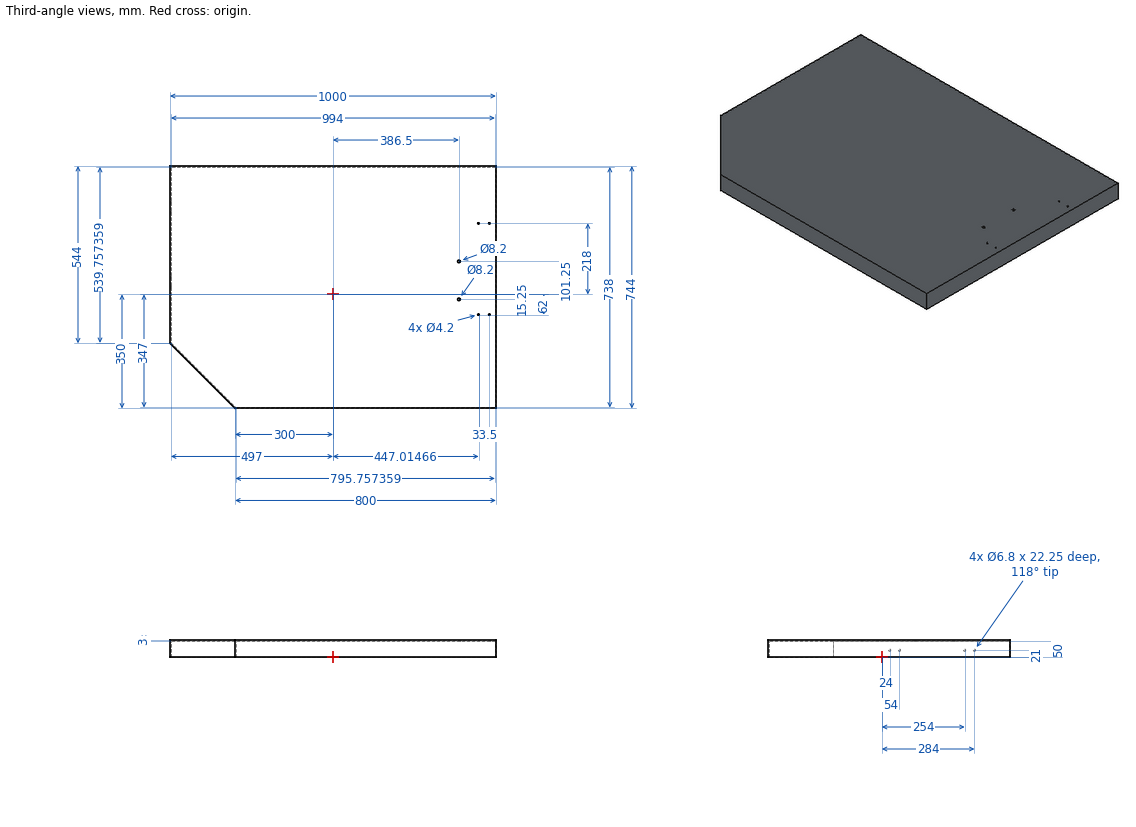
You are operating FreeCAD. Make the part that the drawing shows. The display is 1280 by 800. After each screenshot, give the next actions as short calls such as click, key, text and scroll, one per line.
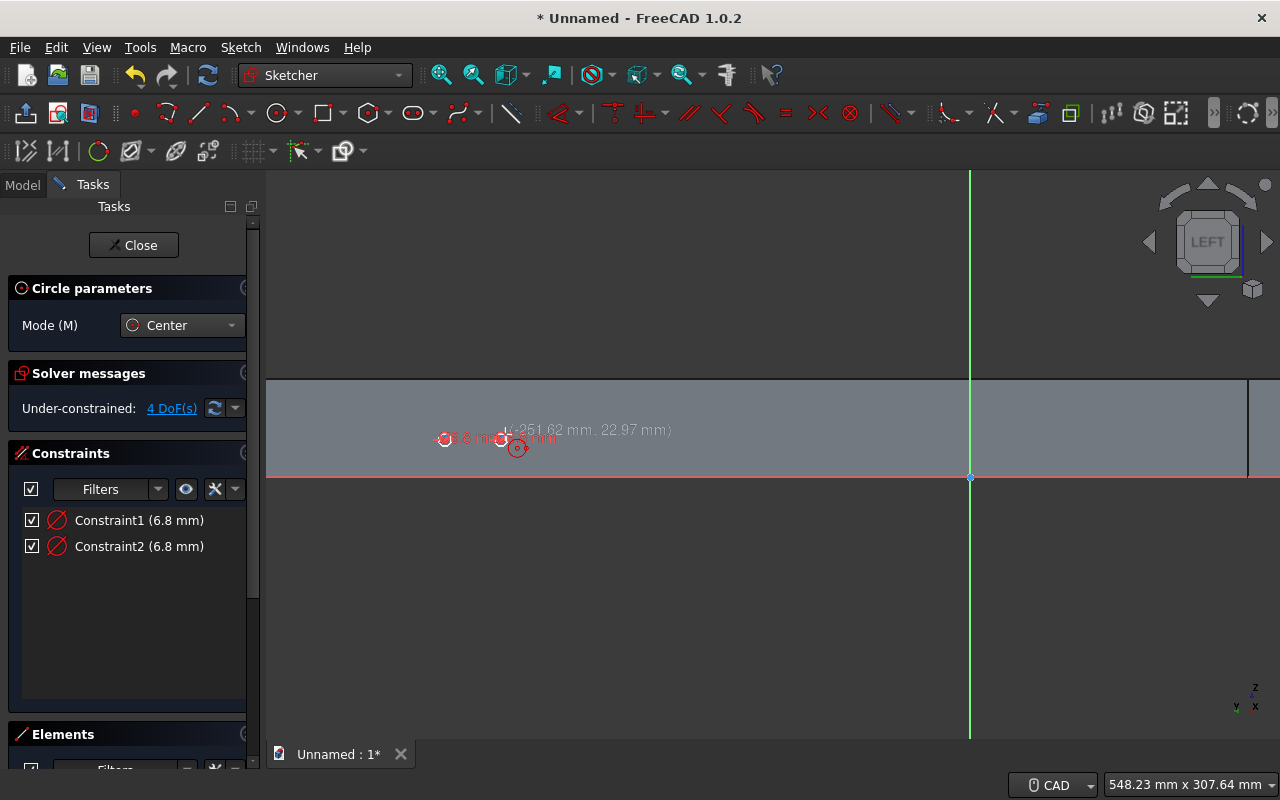
scroll(871, 439, up, 7)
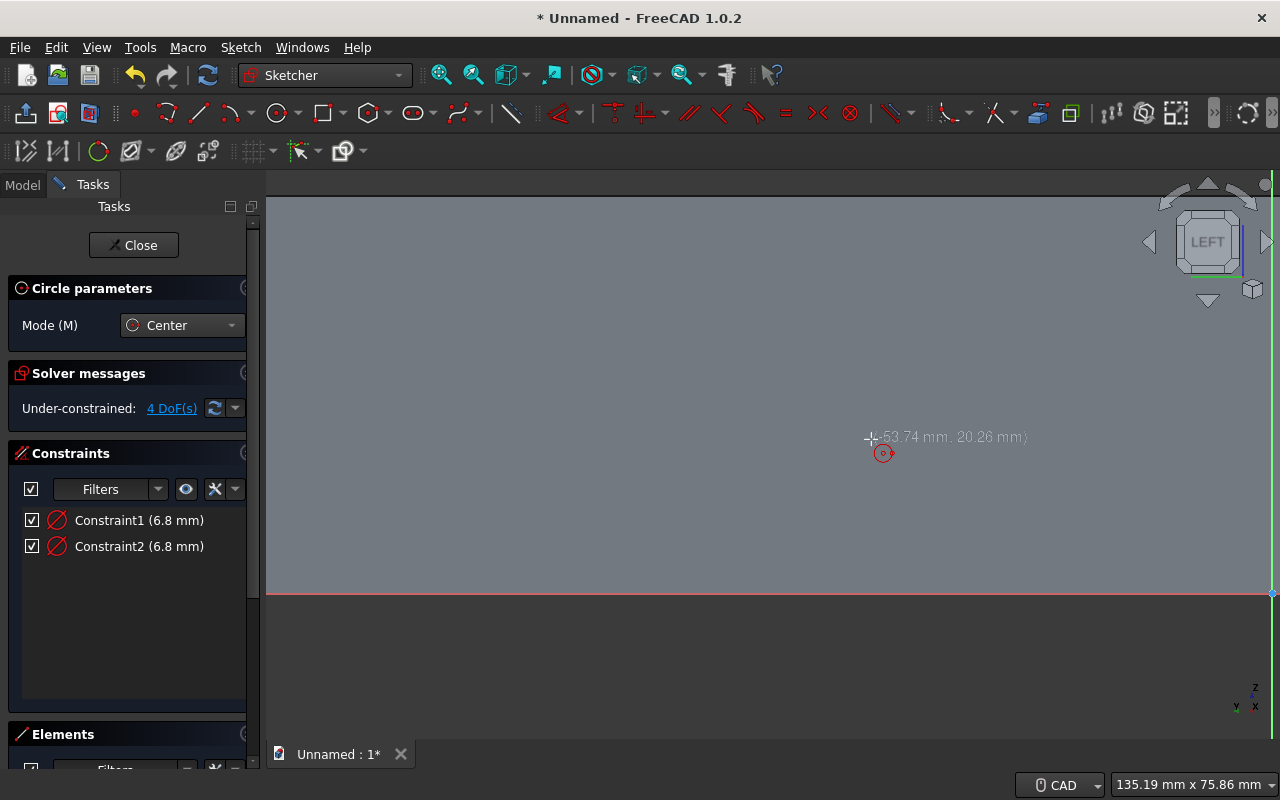
scroll(871, 439, down, 7)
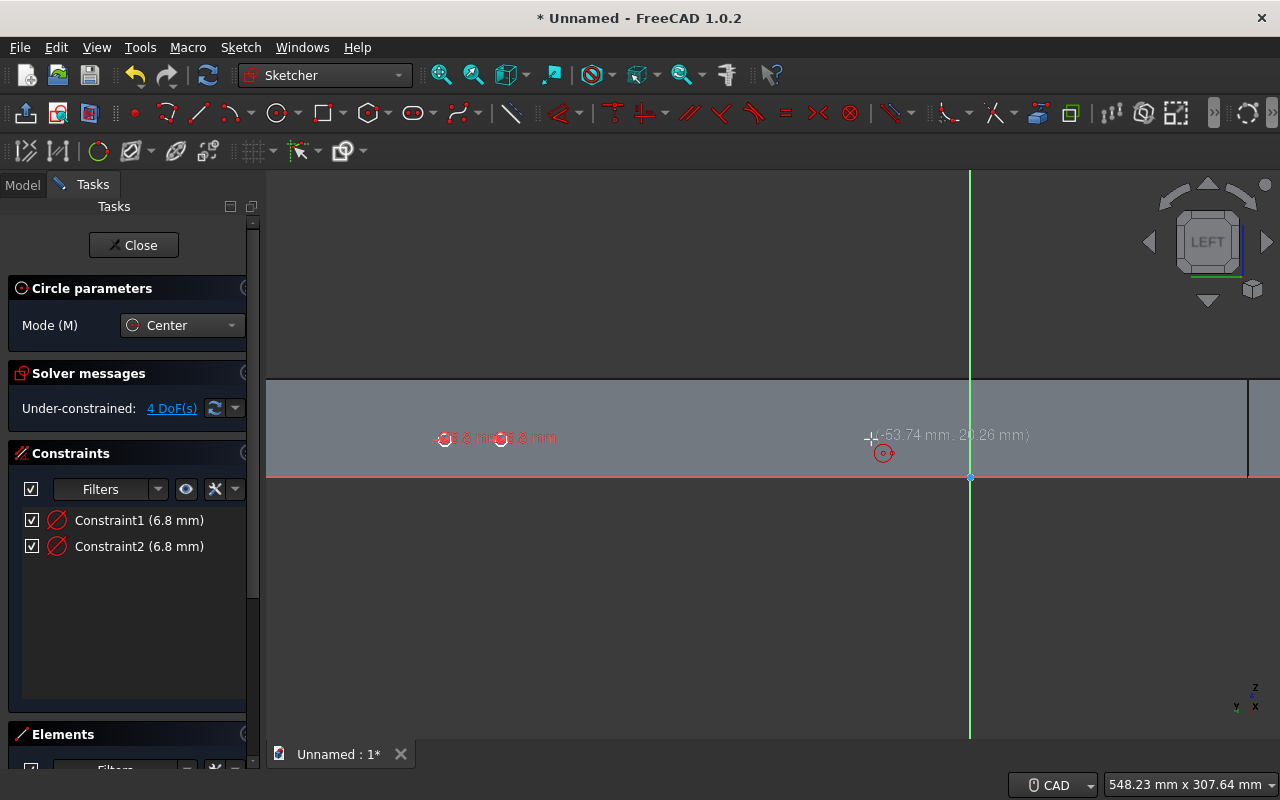
click(871, 439)
move(875, 434)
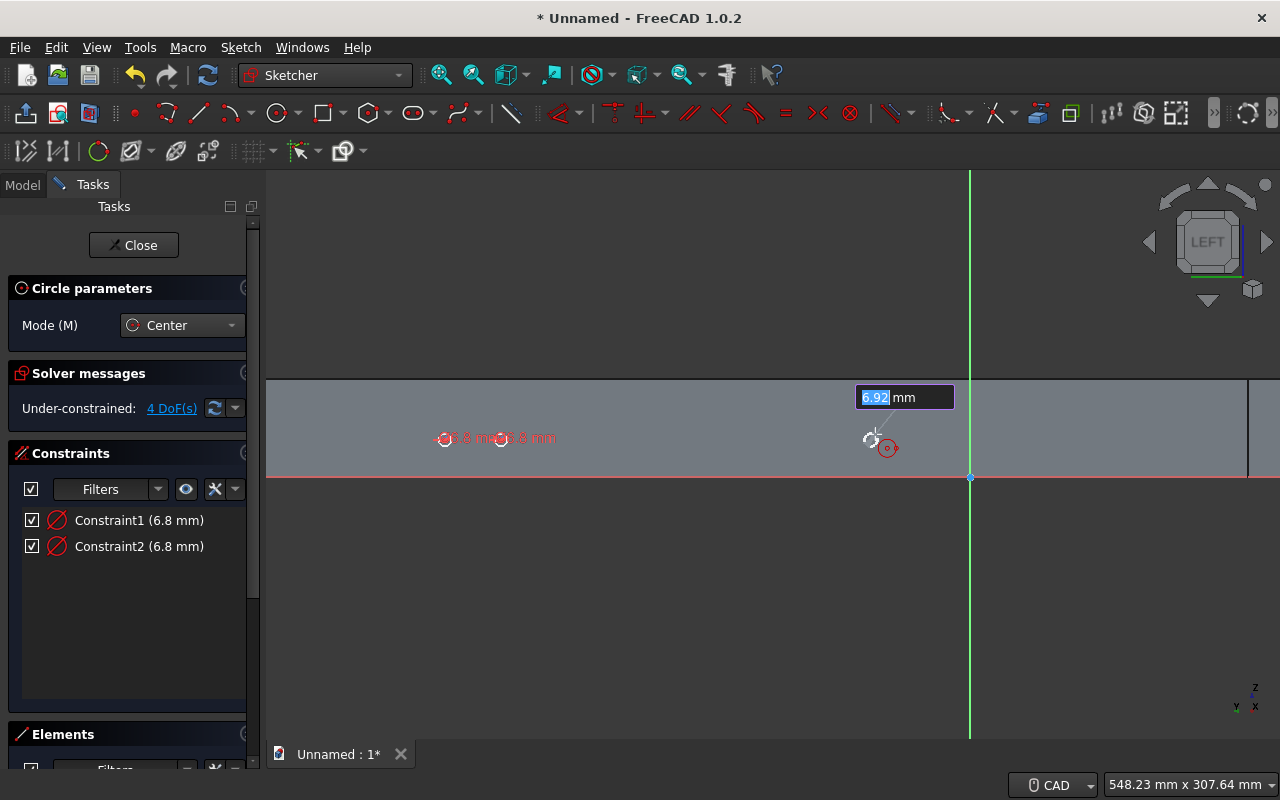
text(6.8)
key(Return)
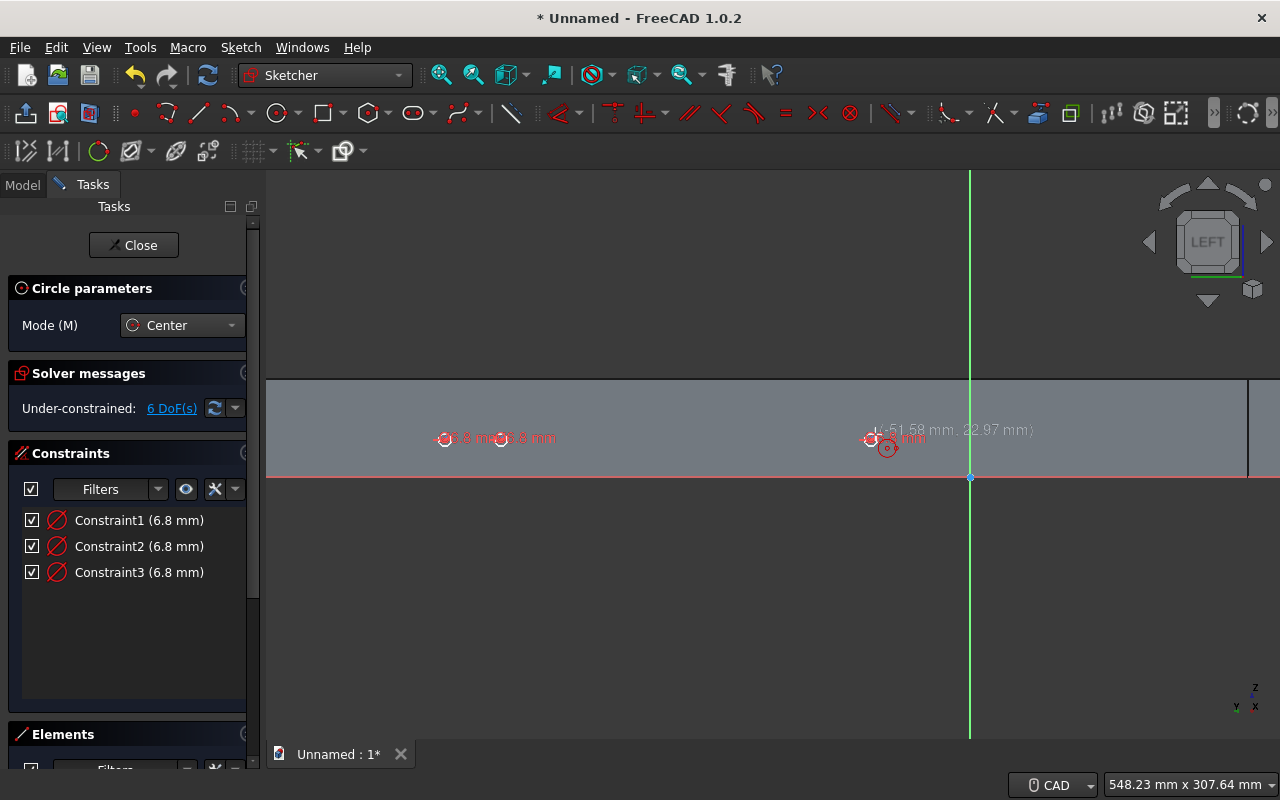
scroll(926, 439, up, 7)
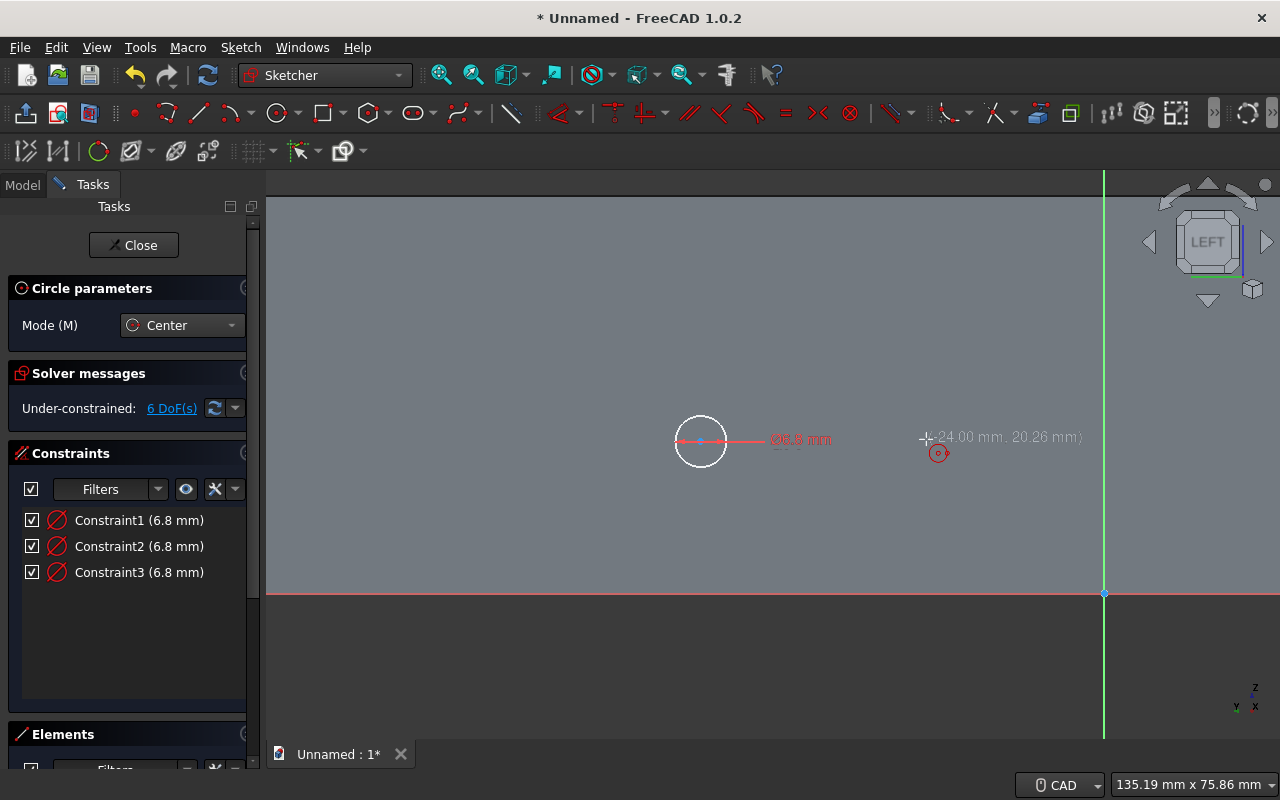
scroll(927, 439, down, 7)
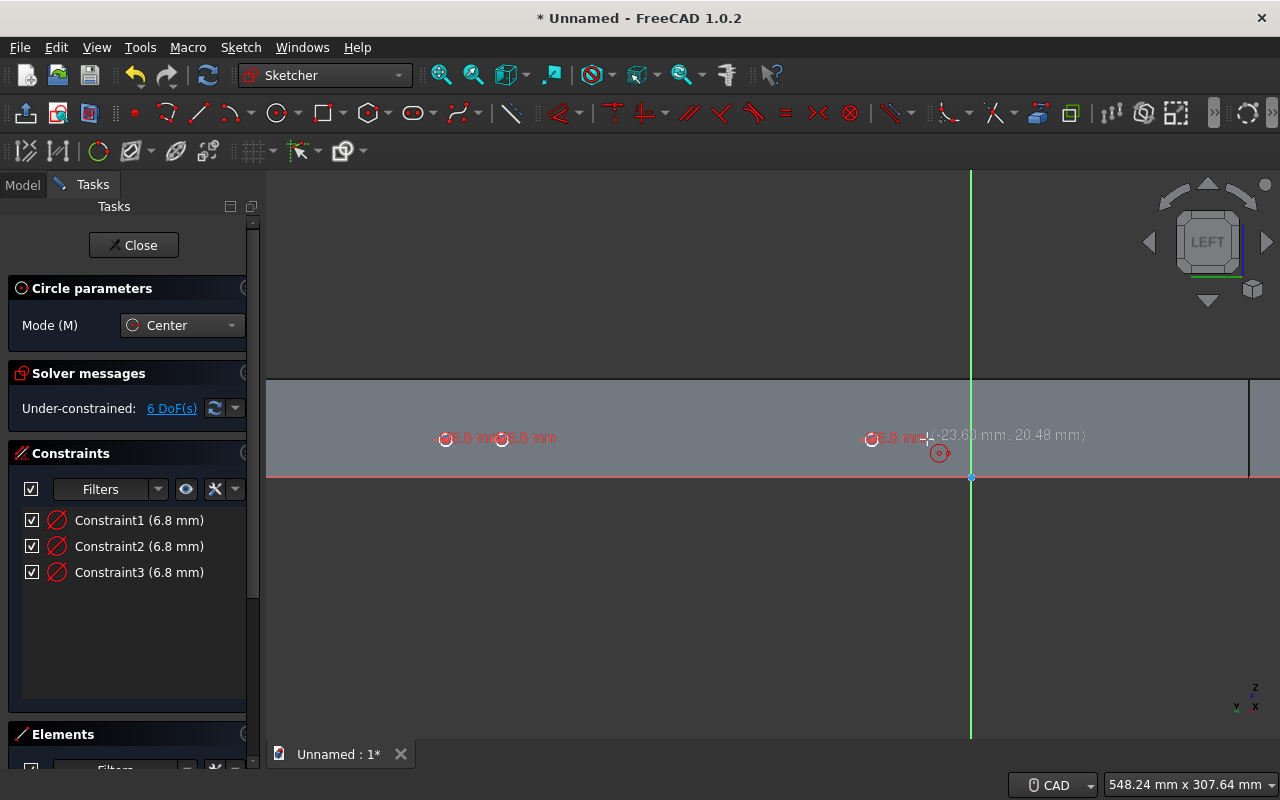
click(927, 439)
move(931, 434)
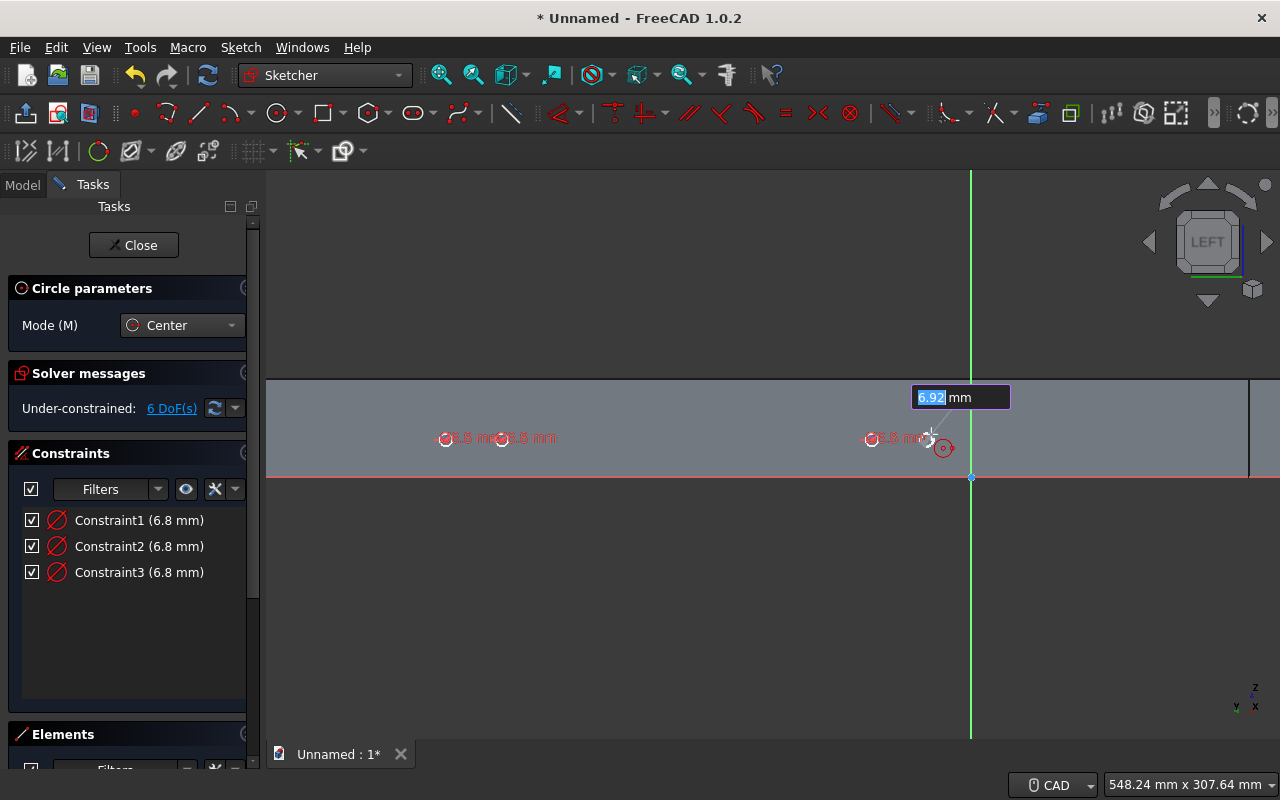
text(6.8)
key(Return)
key(Escape)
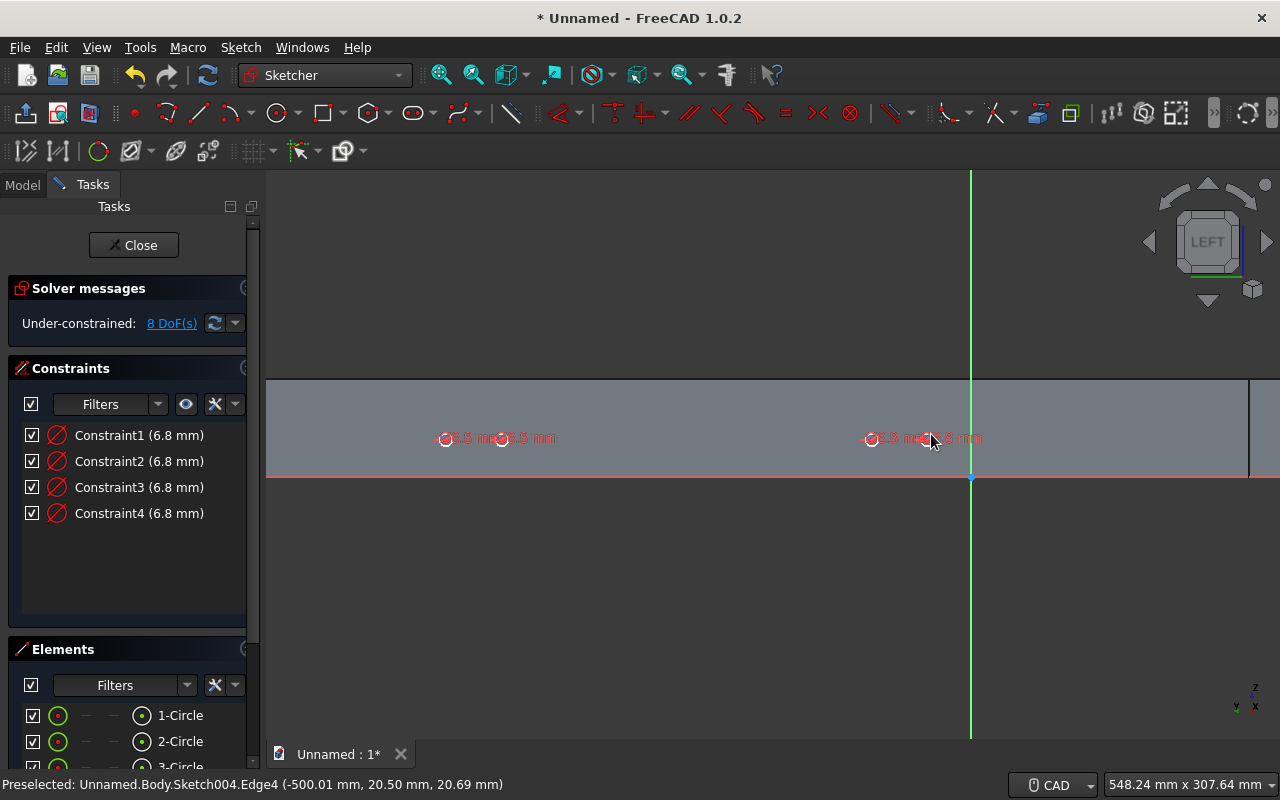
key(d)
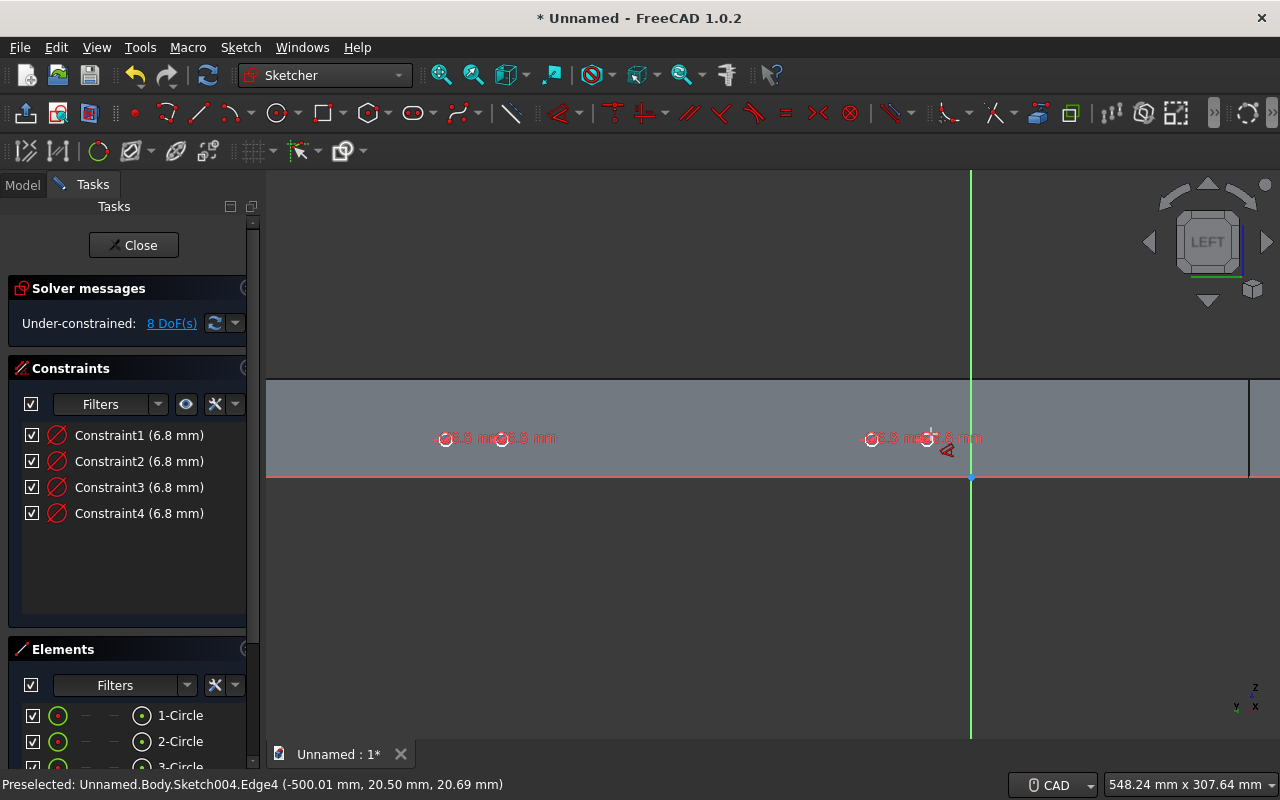
click(446, 440)
click(1005, 459)